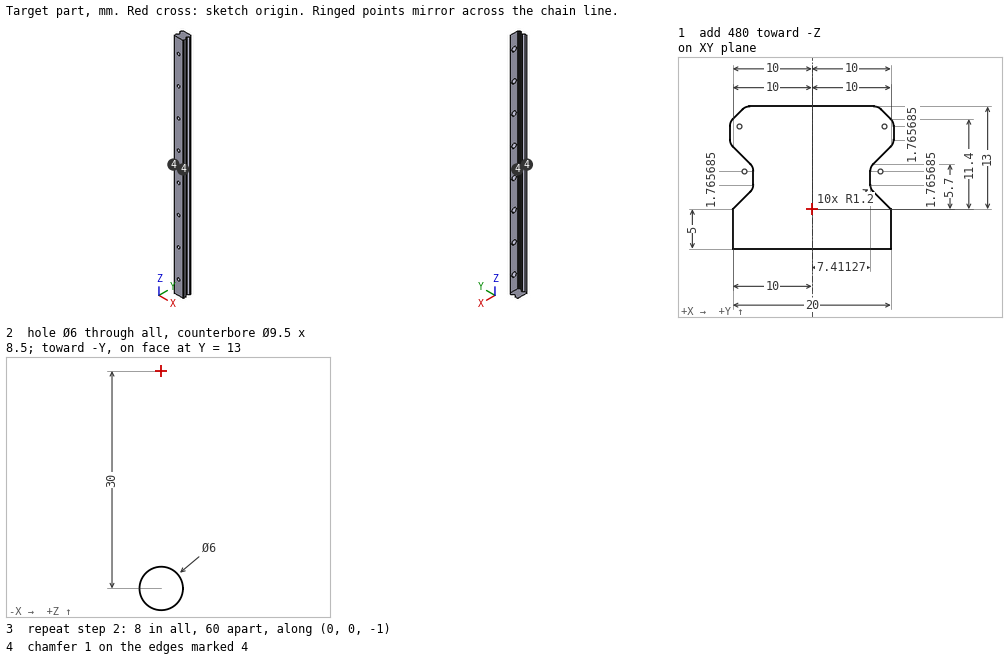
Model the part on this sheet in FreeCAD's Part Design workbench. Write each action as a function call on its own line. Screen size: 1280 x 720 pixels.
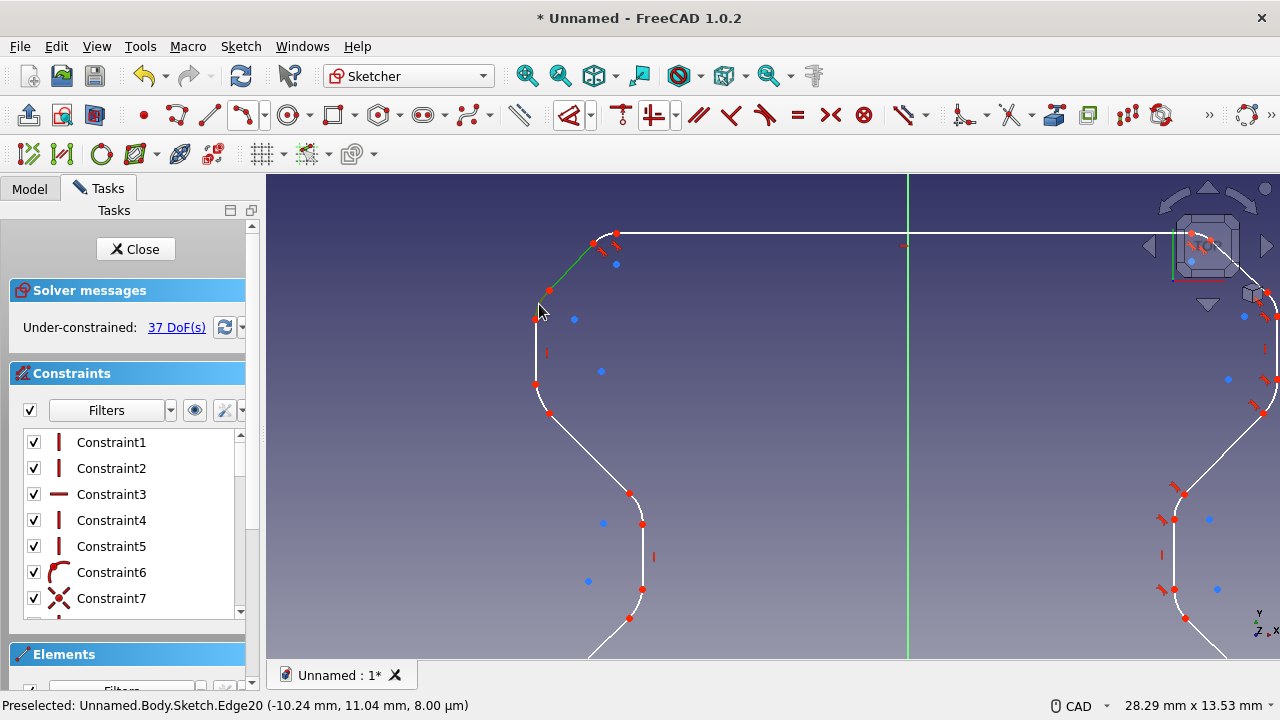
key(t)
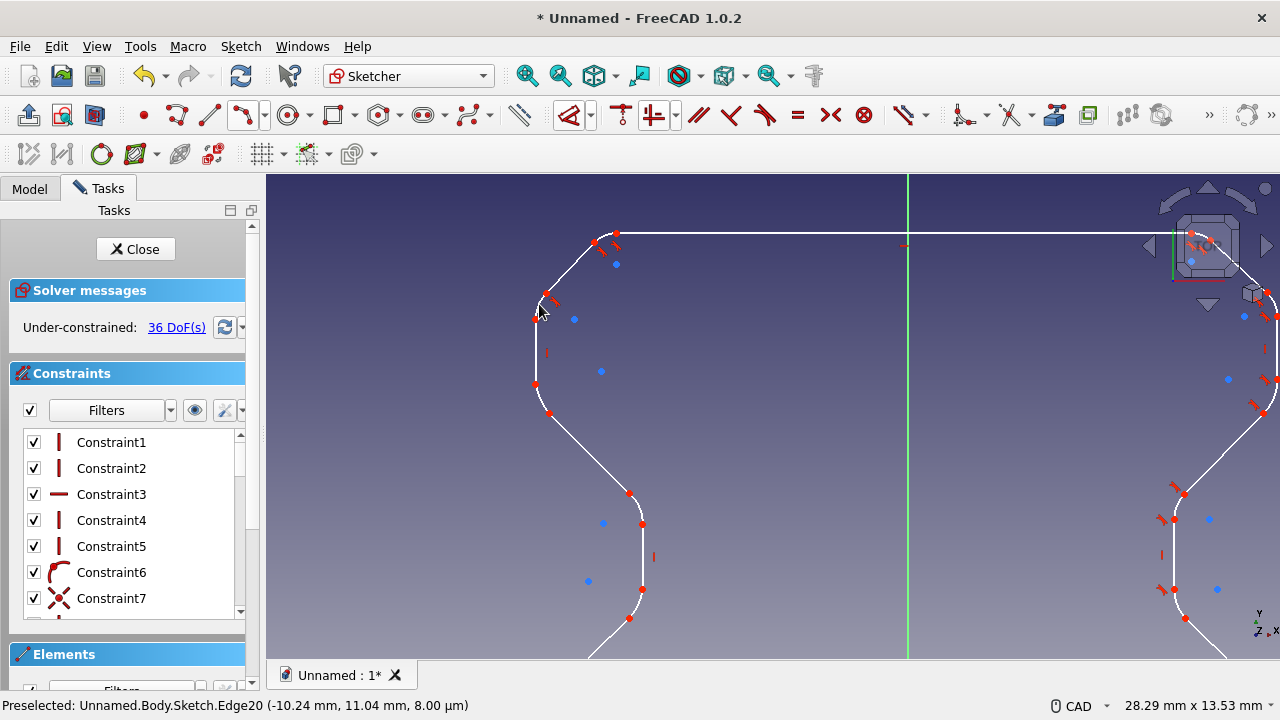
click(536, 339)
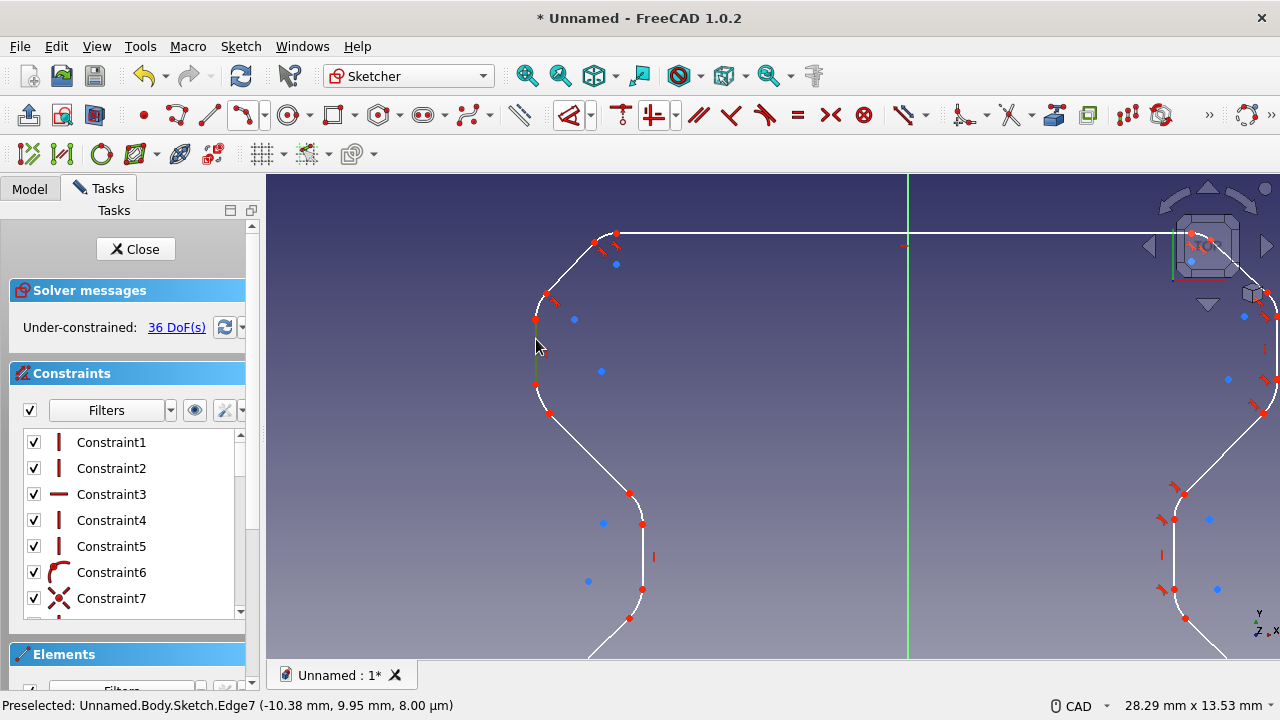
click(539, 306)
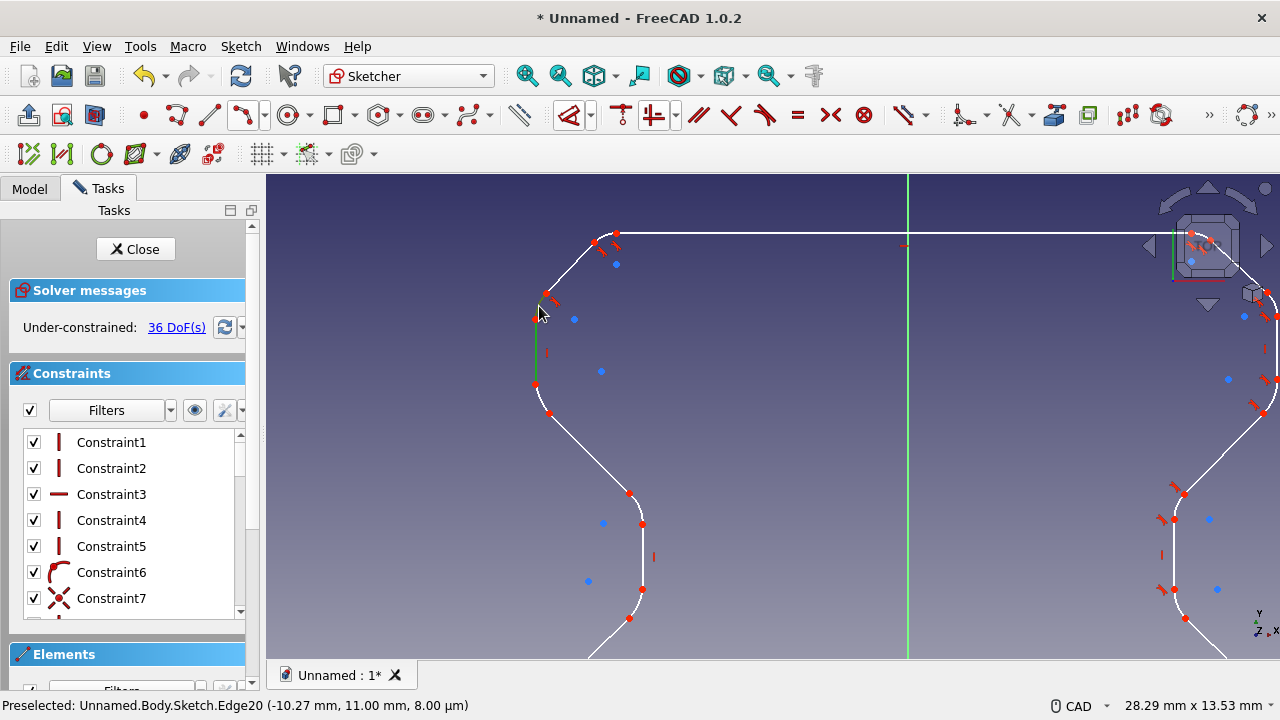
key(t)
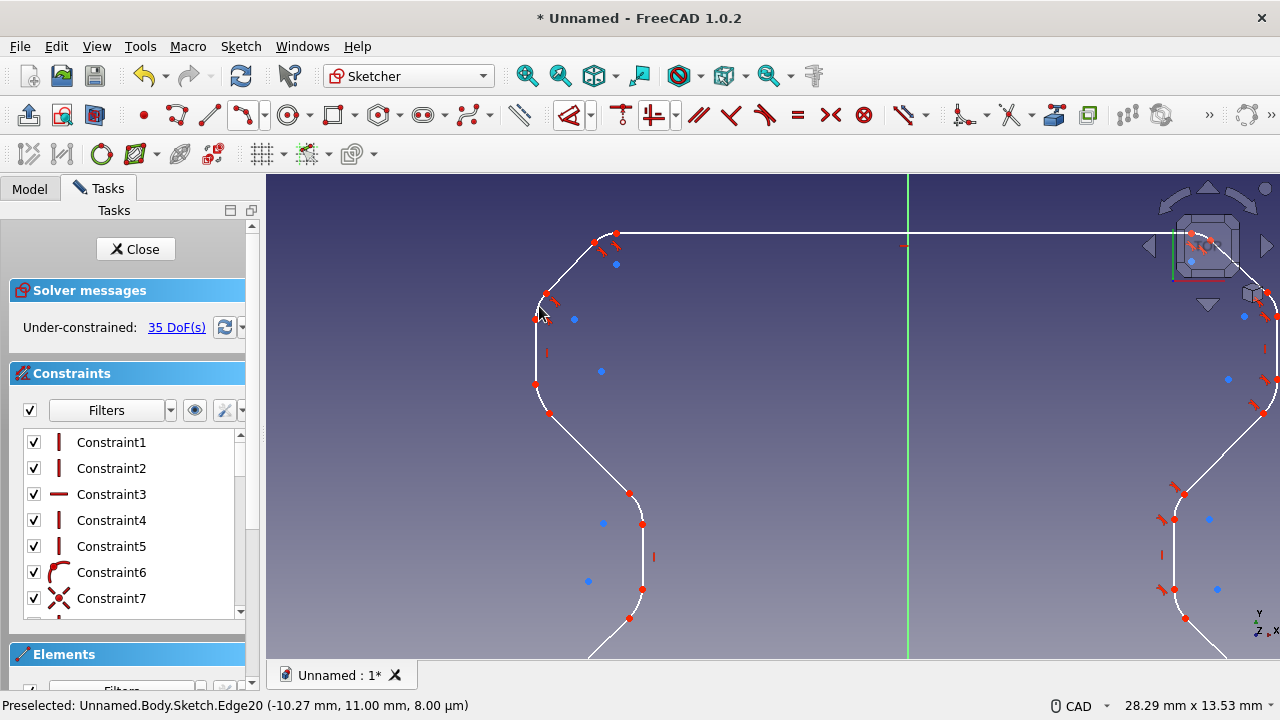
click(536, 339)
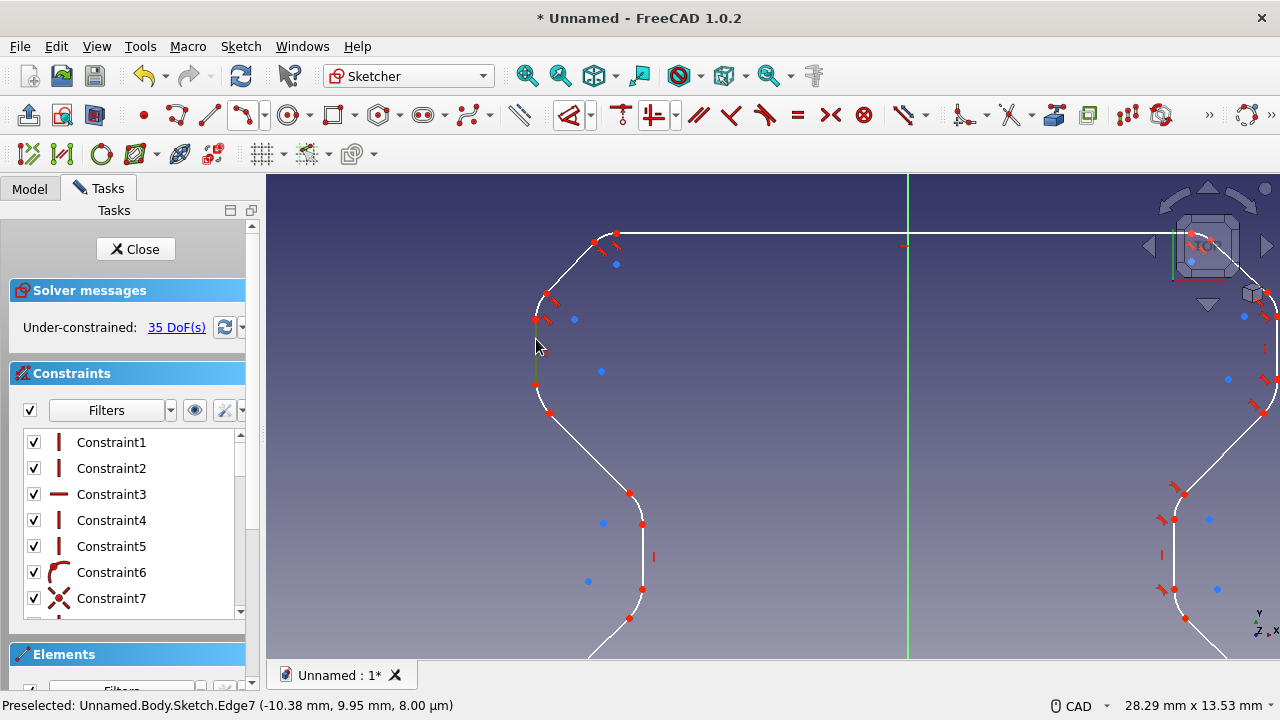
scroll(538, 394, up, 2)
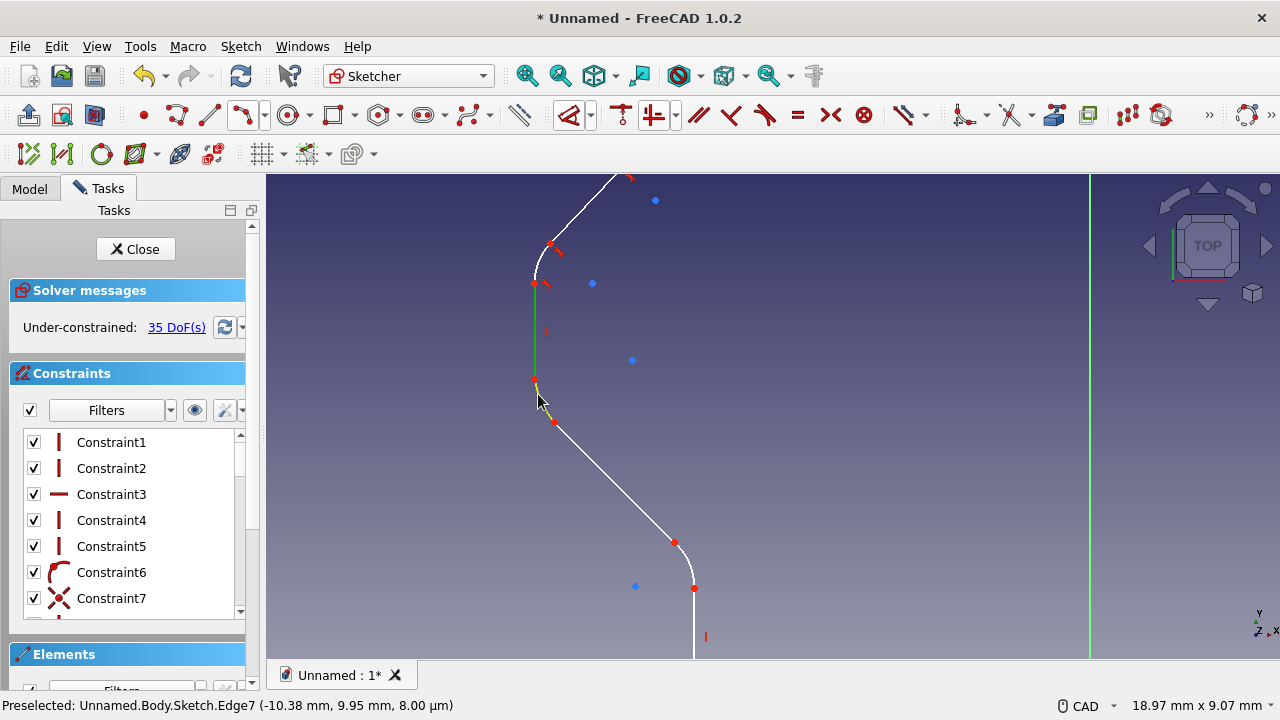
click(538, 393)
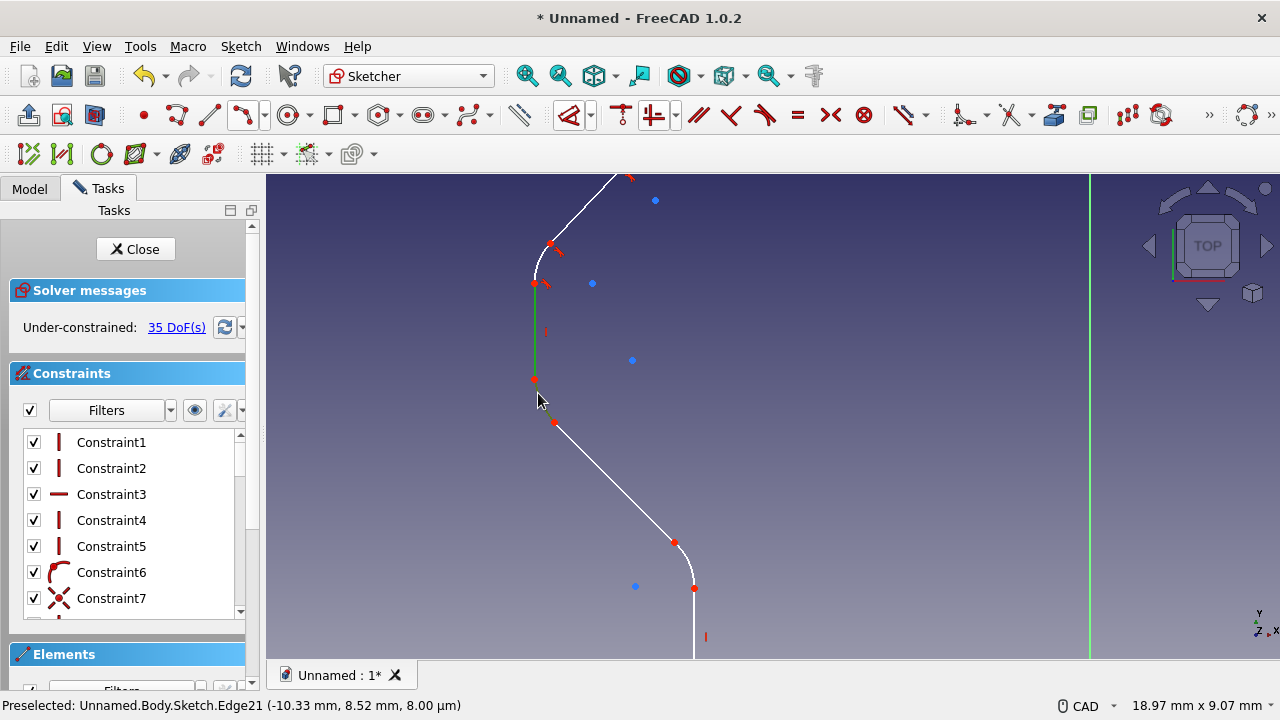
key(t)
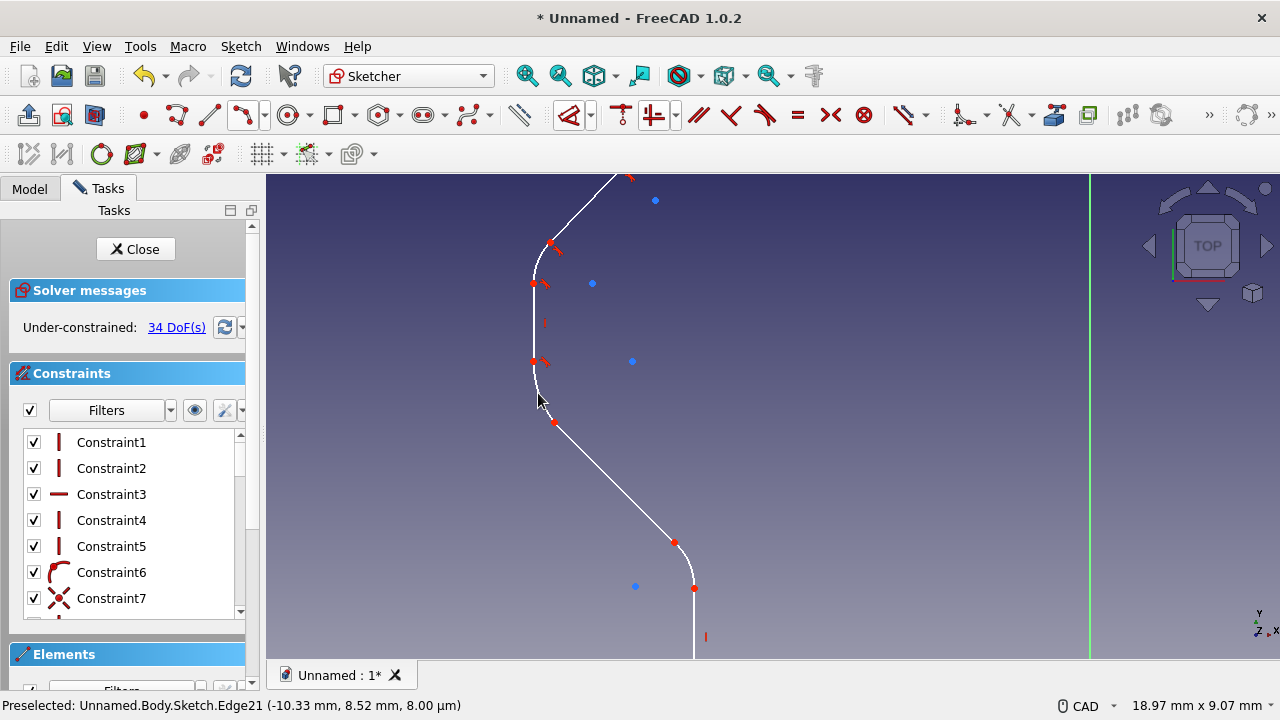
click(590, 458)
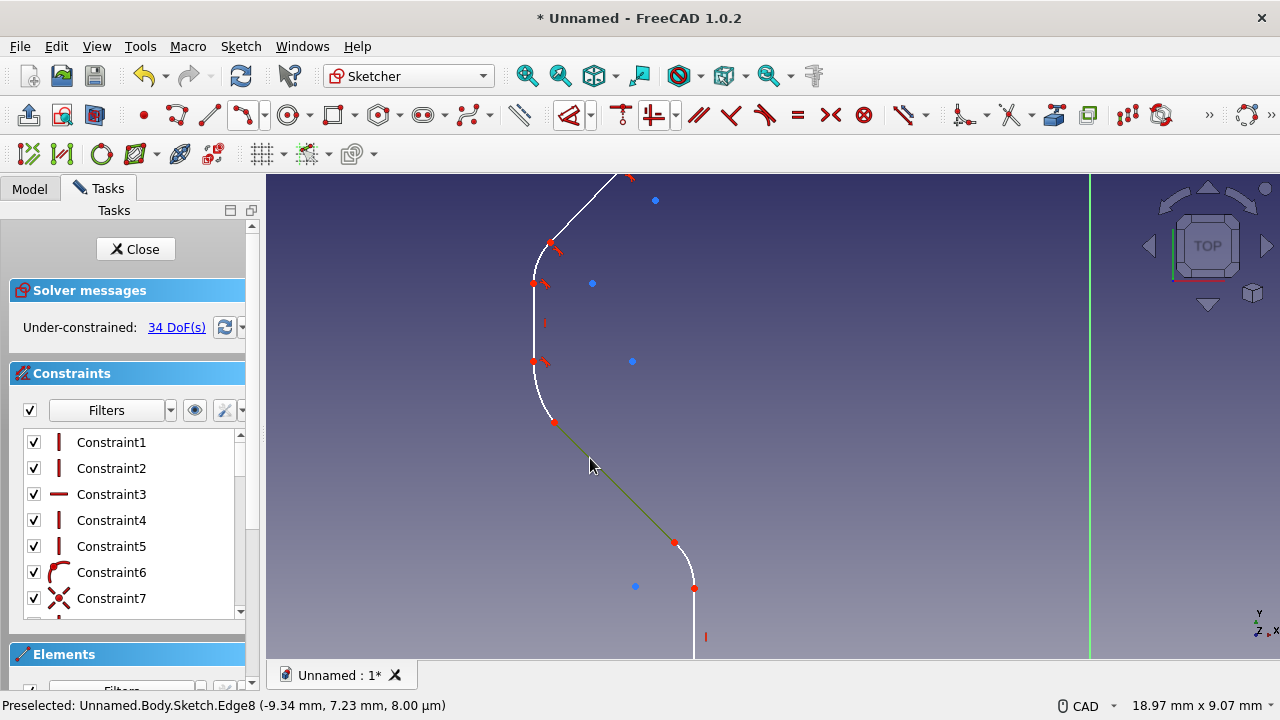
click(536, 381)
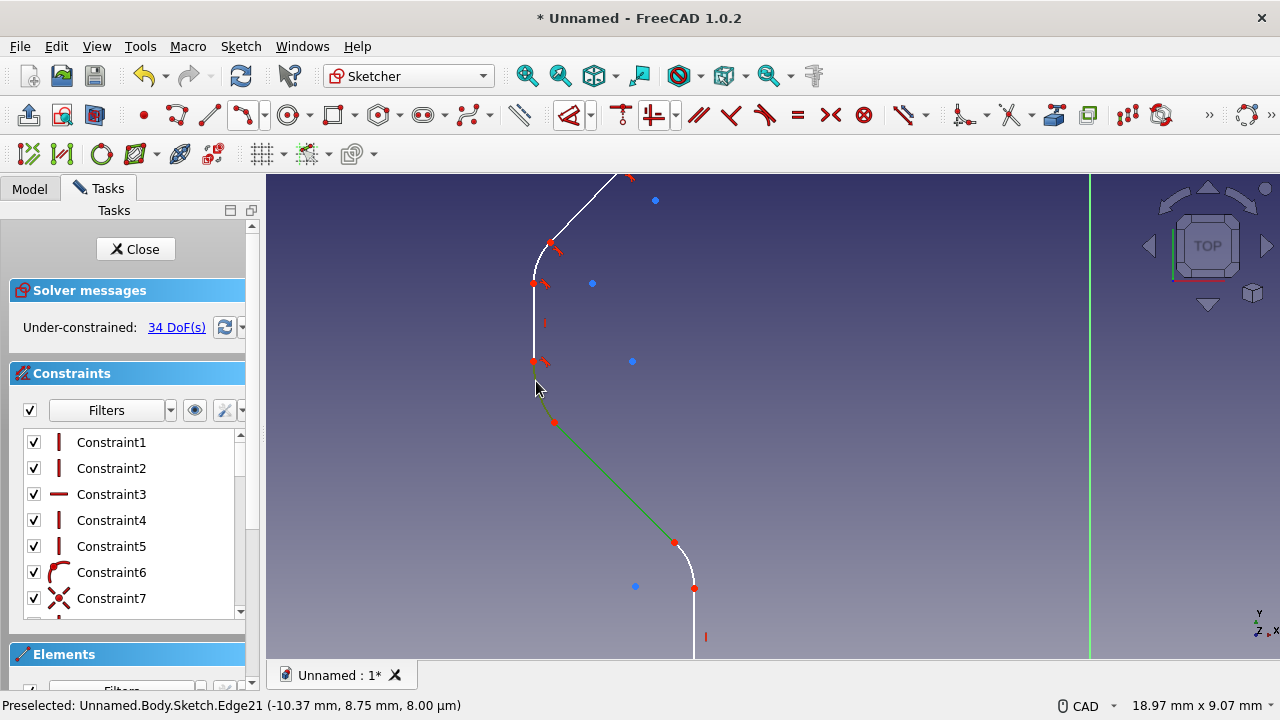
key(t)